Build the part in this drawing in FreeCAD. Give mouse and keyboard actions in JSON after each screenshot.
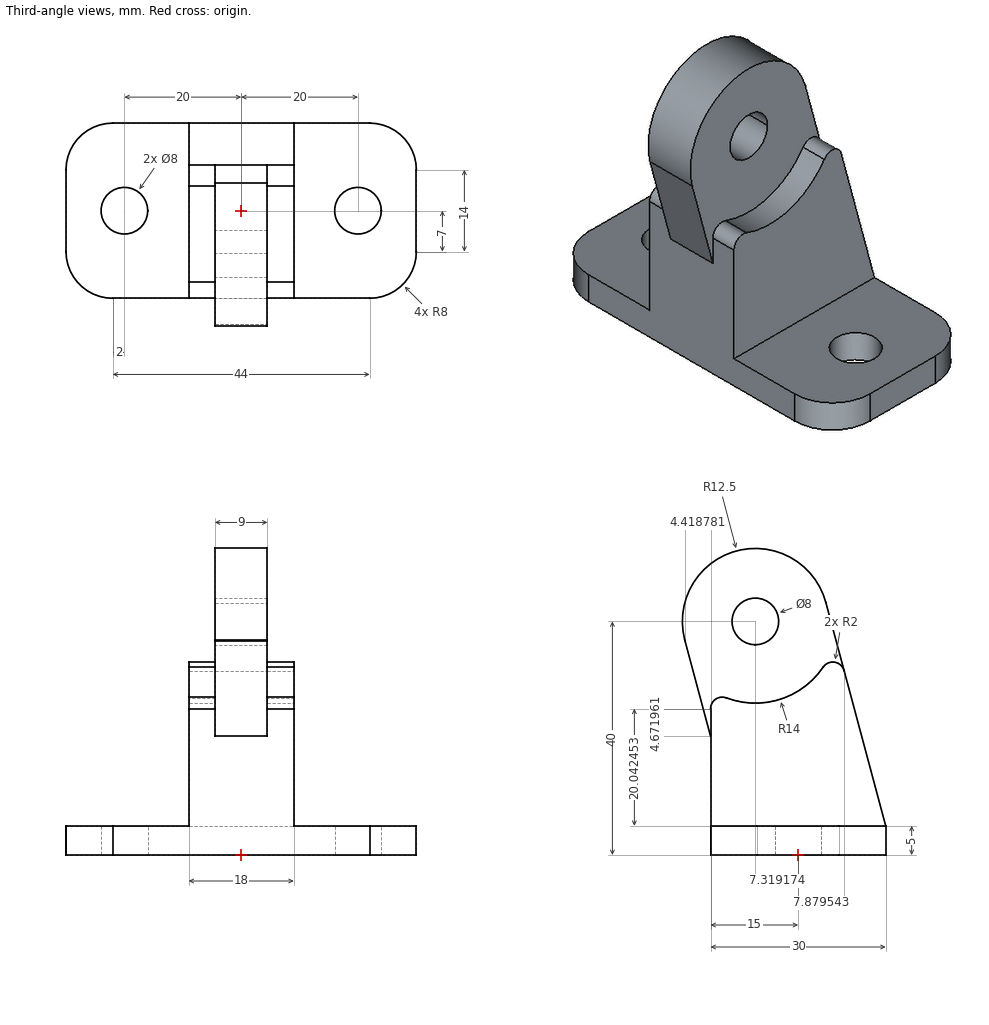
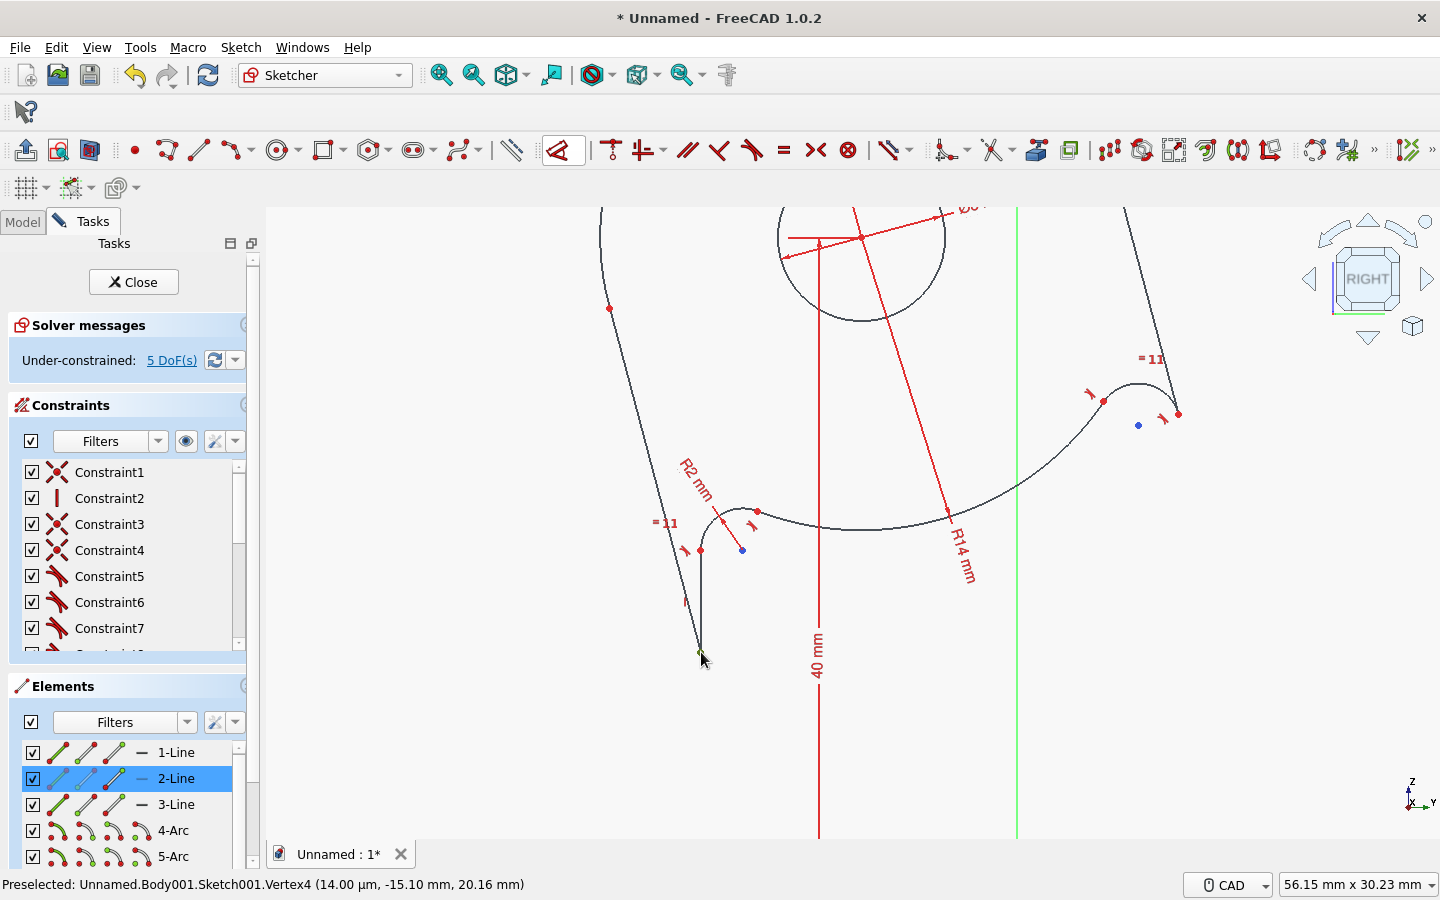
{"action": "key", "text": "l"}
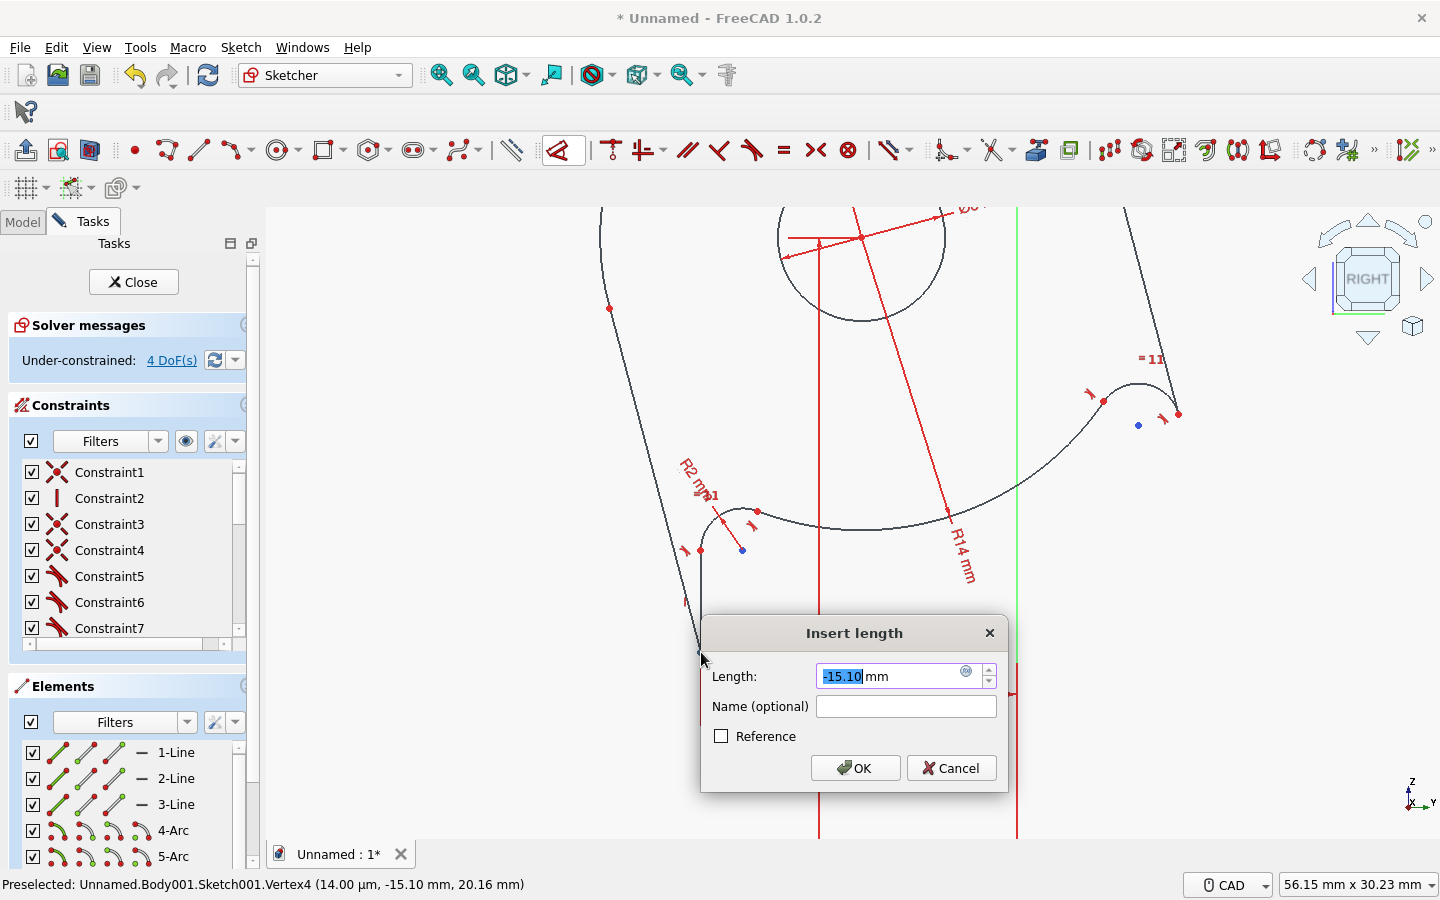
{"action": "type", "text": "-15"}
{"action": "key", "text": "Return"}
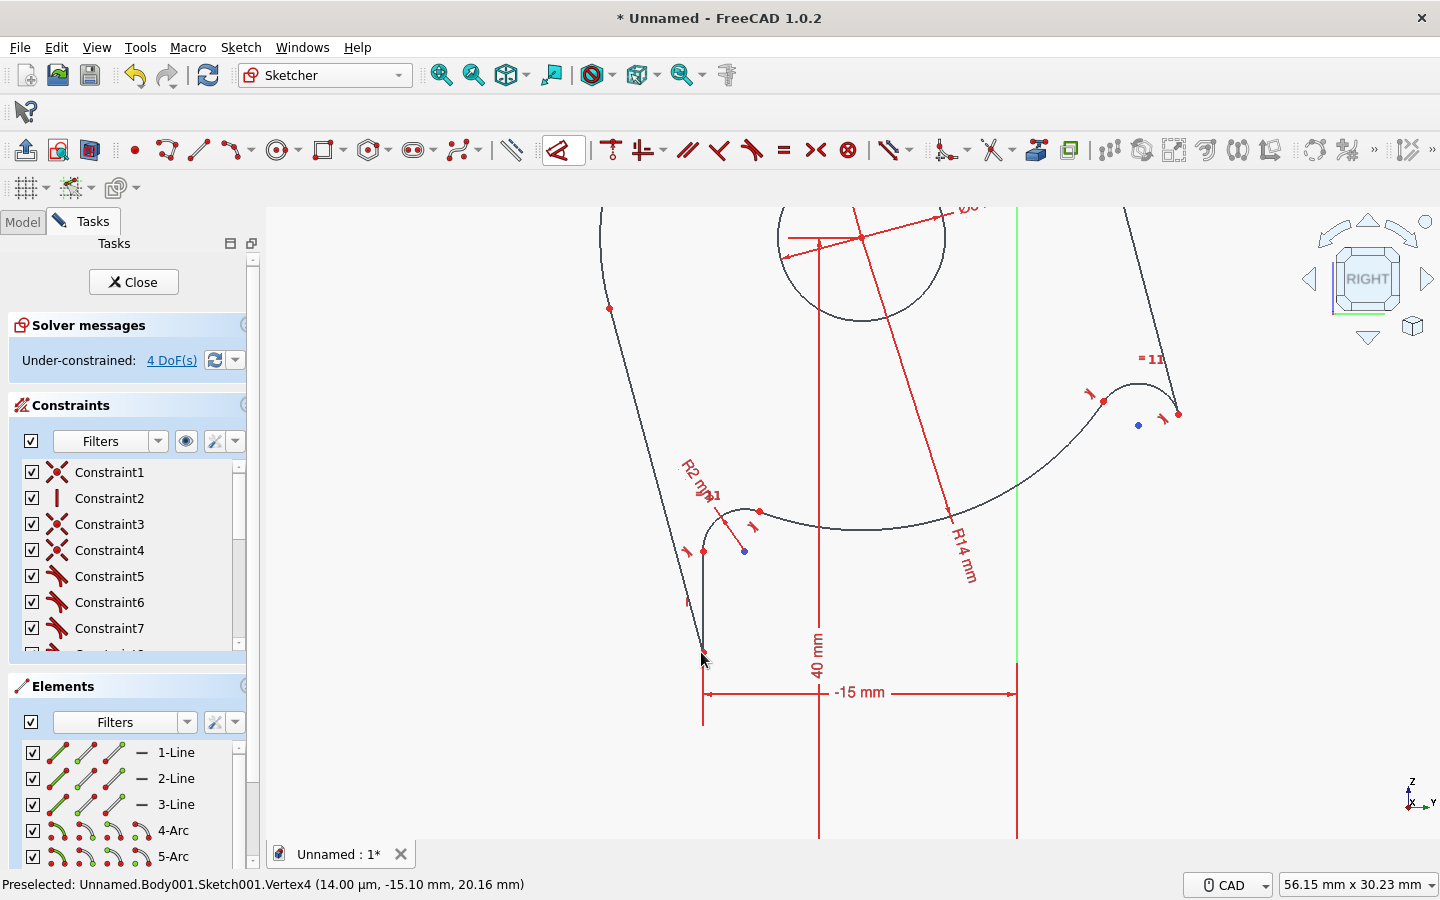
{"action": "left_click", "coordinate": [703, 581]}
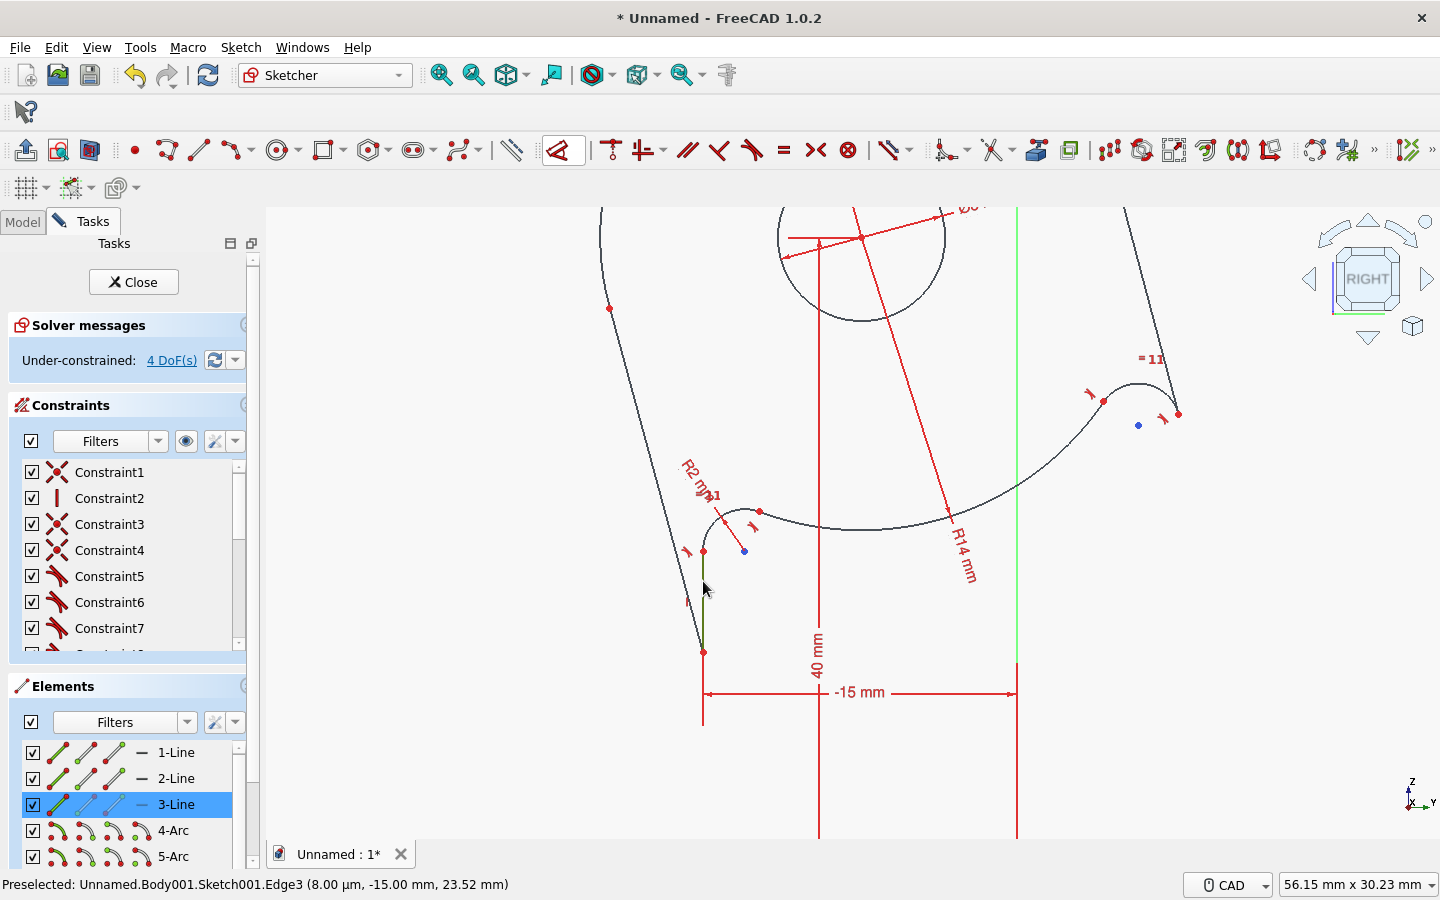
{"action": "key", "text": "i"}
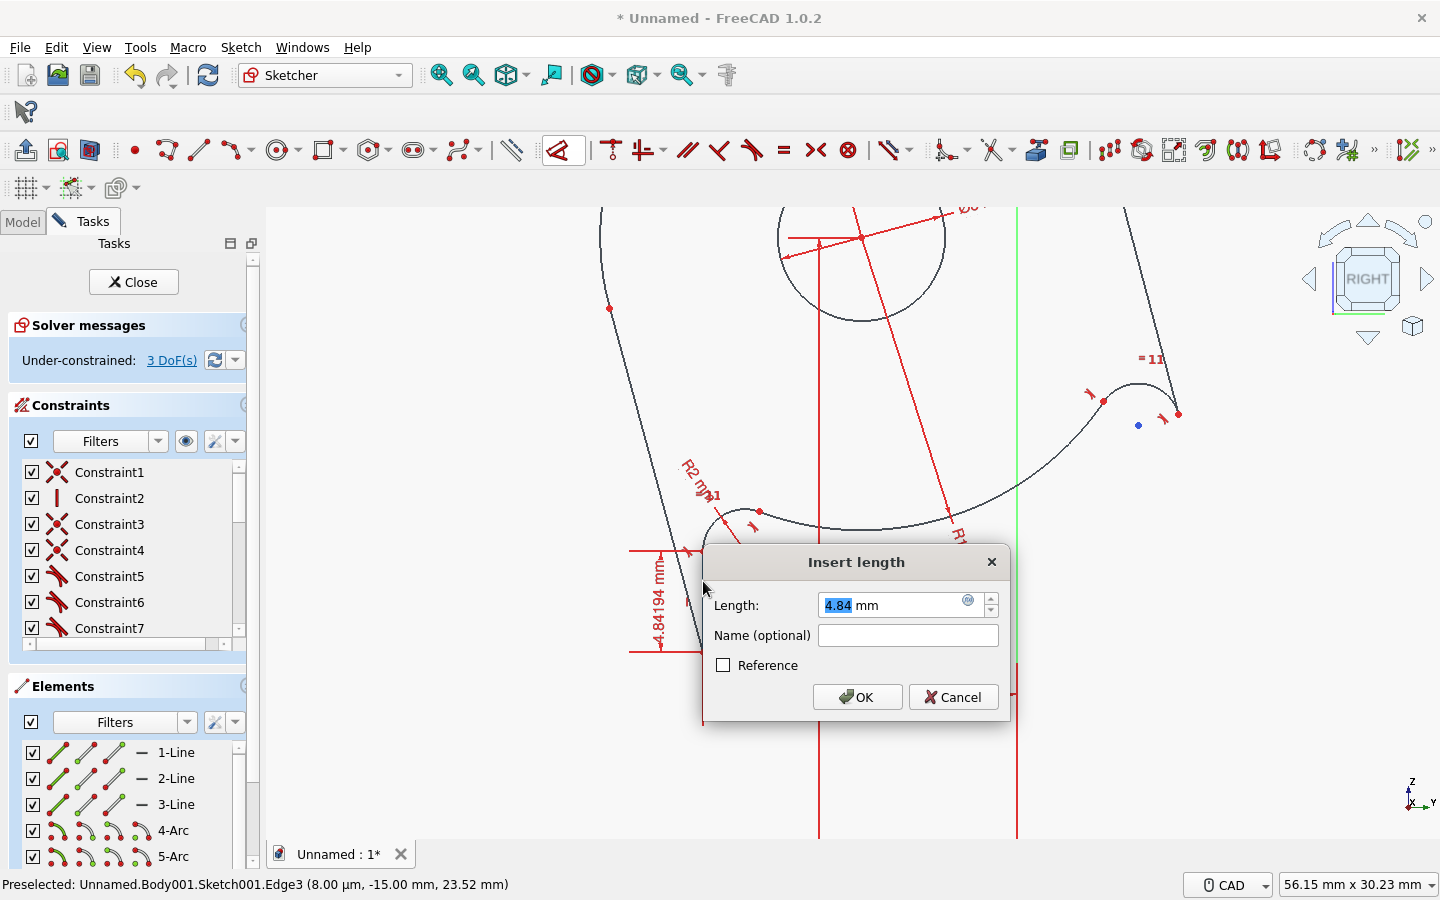
{"action": "type", "text": "4.671961"}
{"action": "key", "text": "Return"}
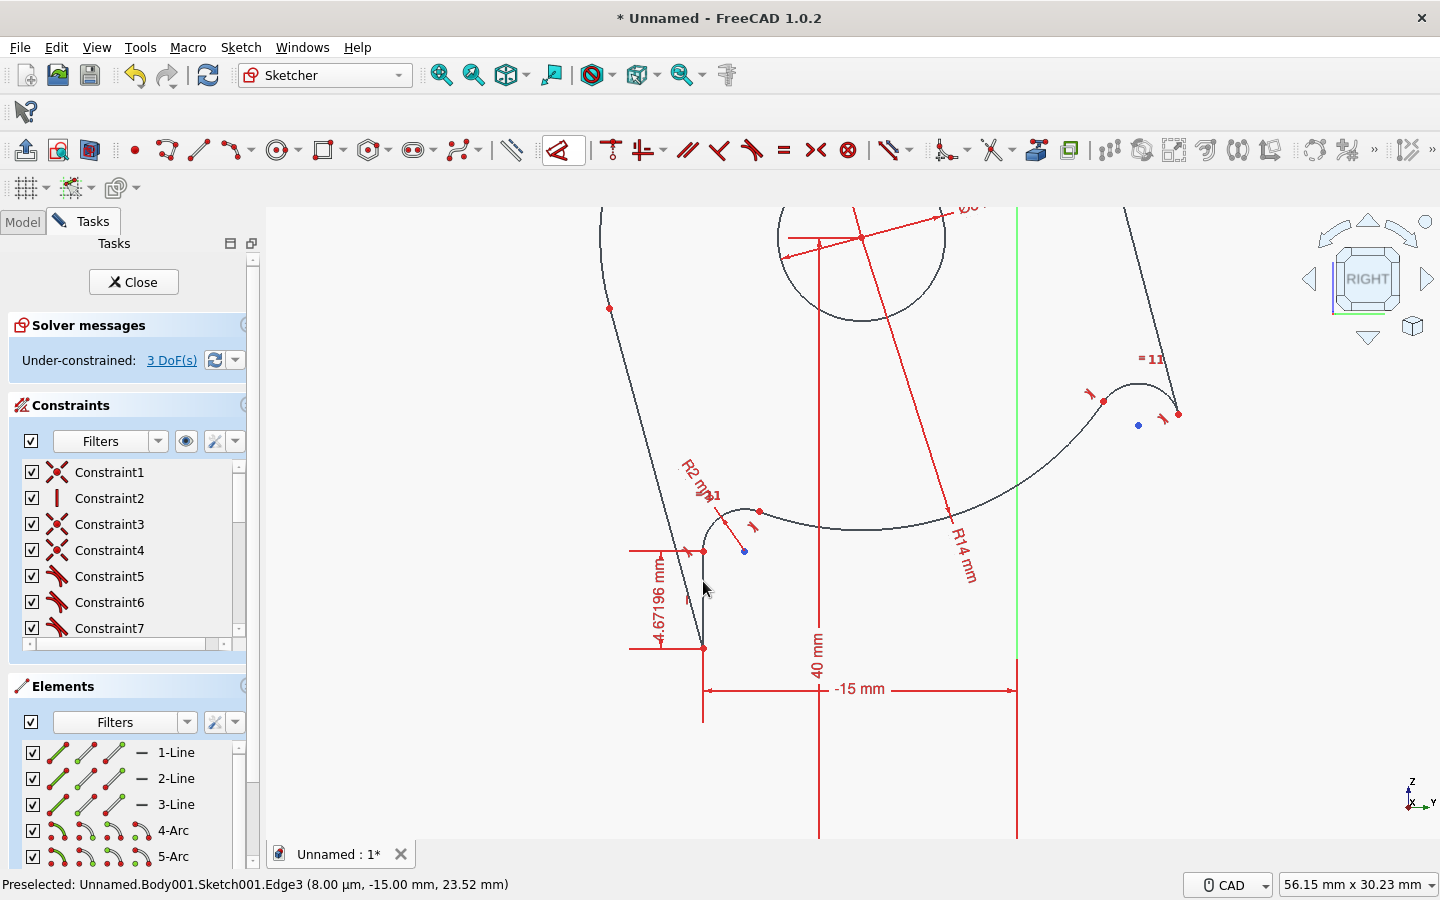
{"action": "left_click", "coordinate": [862, 238]}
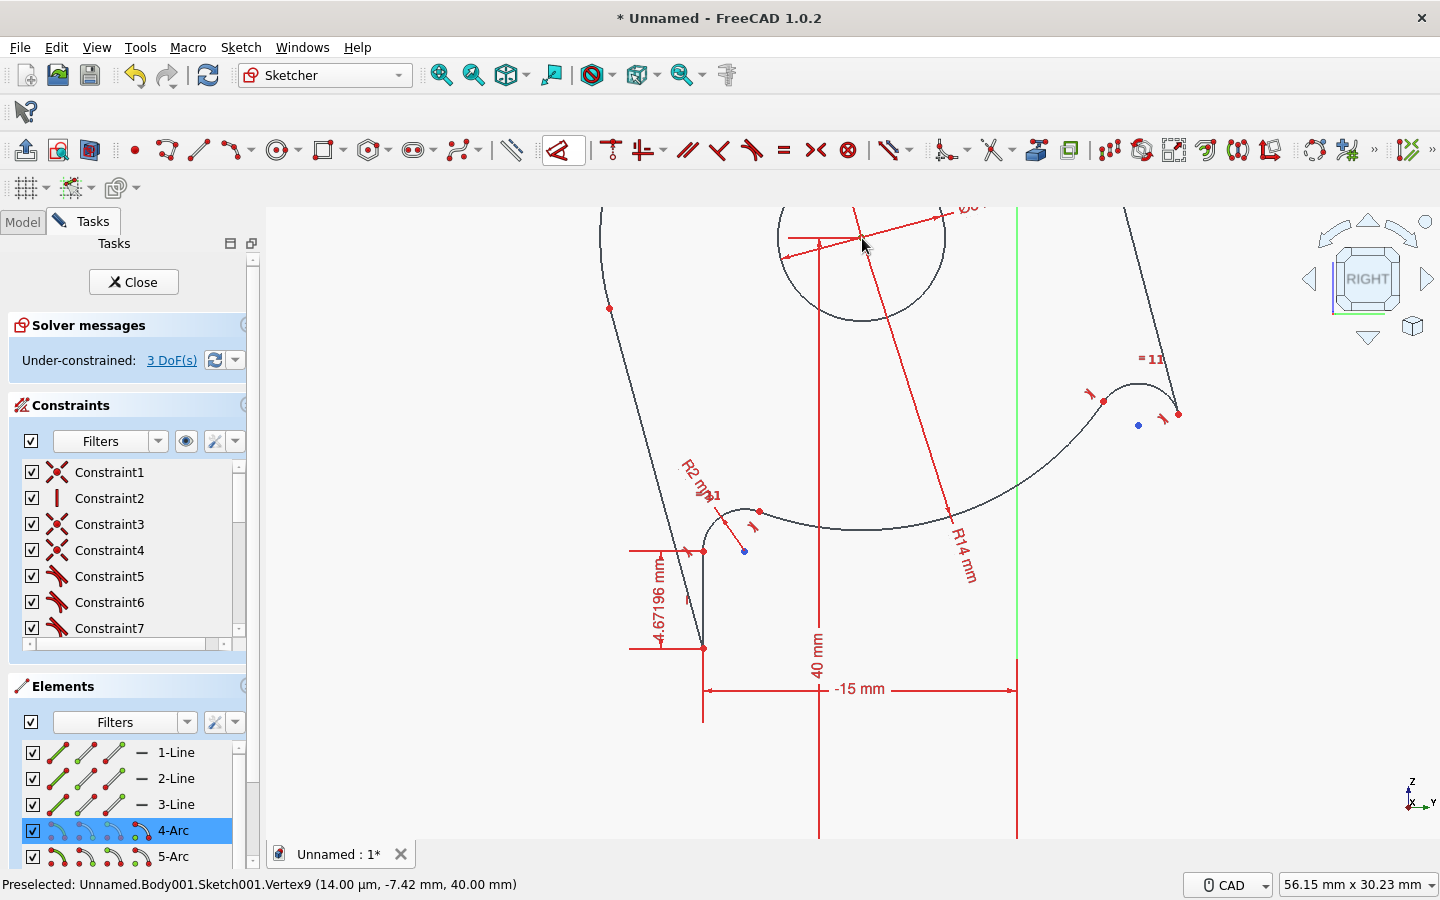
{"action": "left_click", "coordinate": [580, 150]}